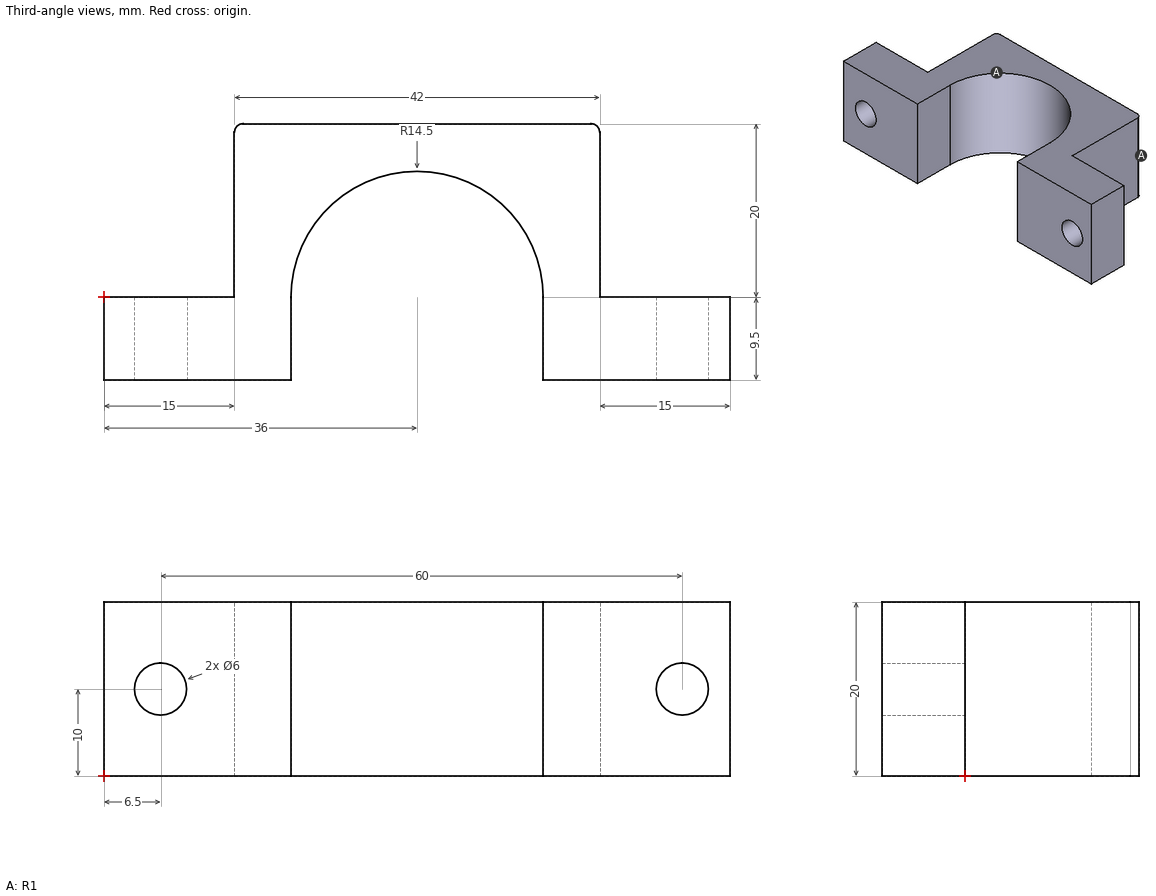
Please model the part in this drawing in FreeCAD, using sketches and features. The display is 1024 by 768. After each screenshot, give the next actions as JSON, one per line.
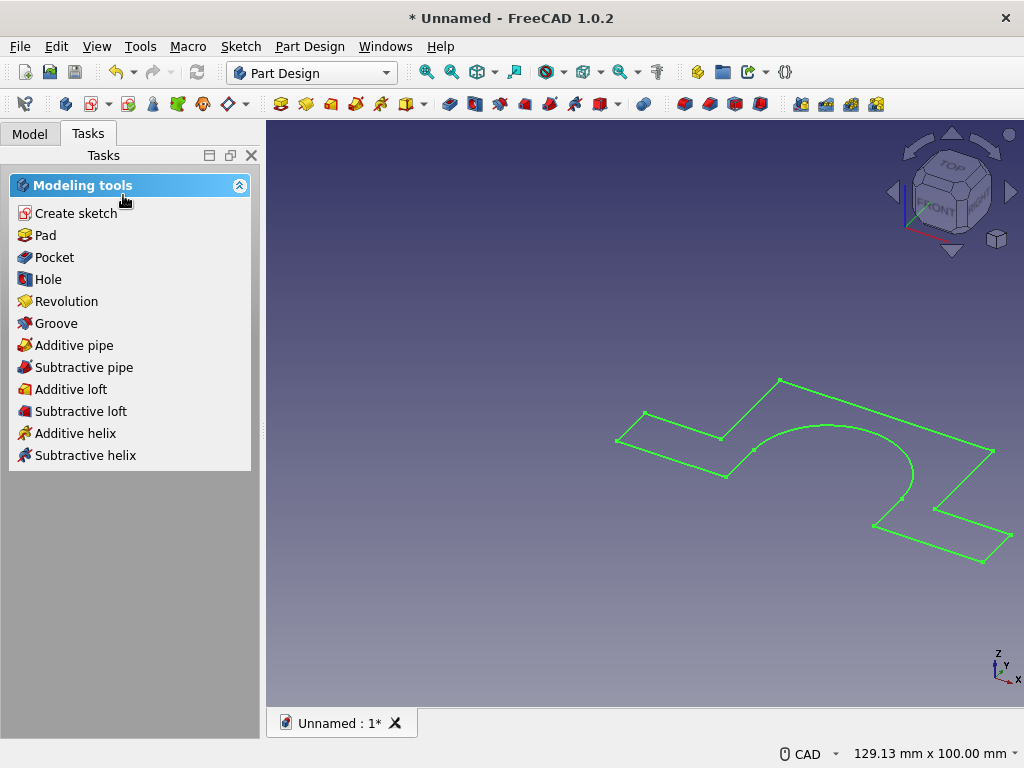
{"action": "left_click", "coordinate": [281, 104]}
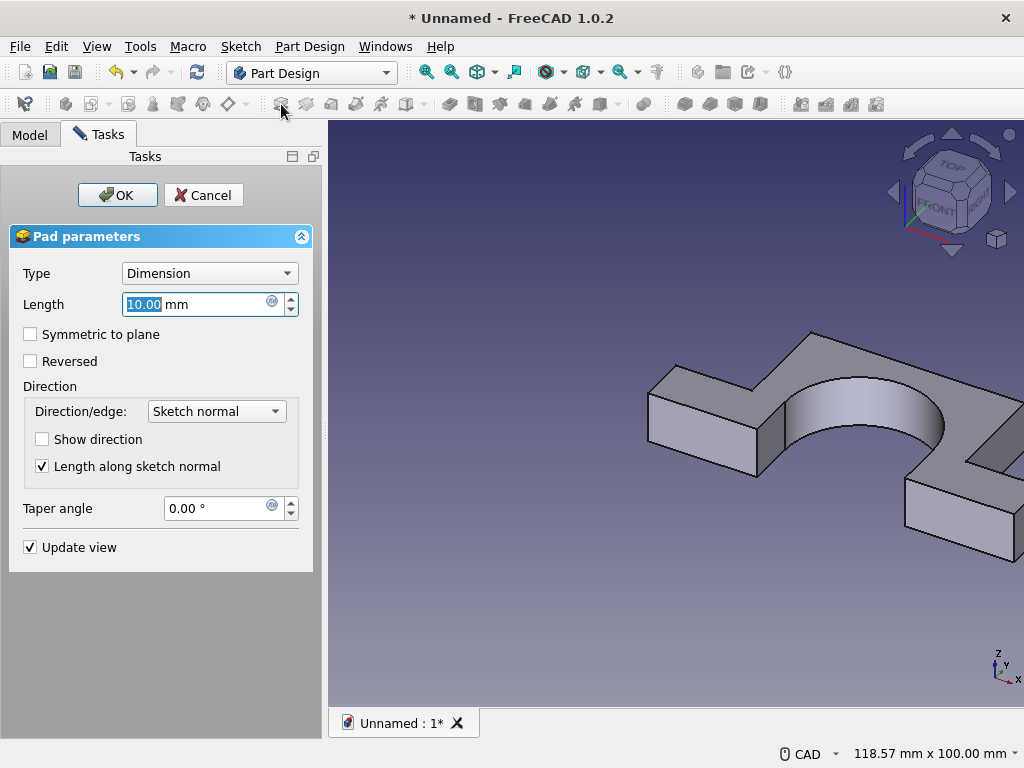
{"action": "type", "text": "20"}
{"action": "key", "text": "Tab"}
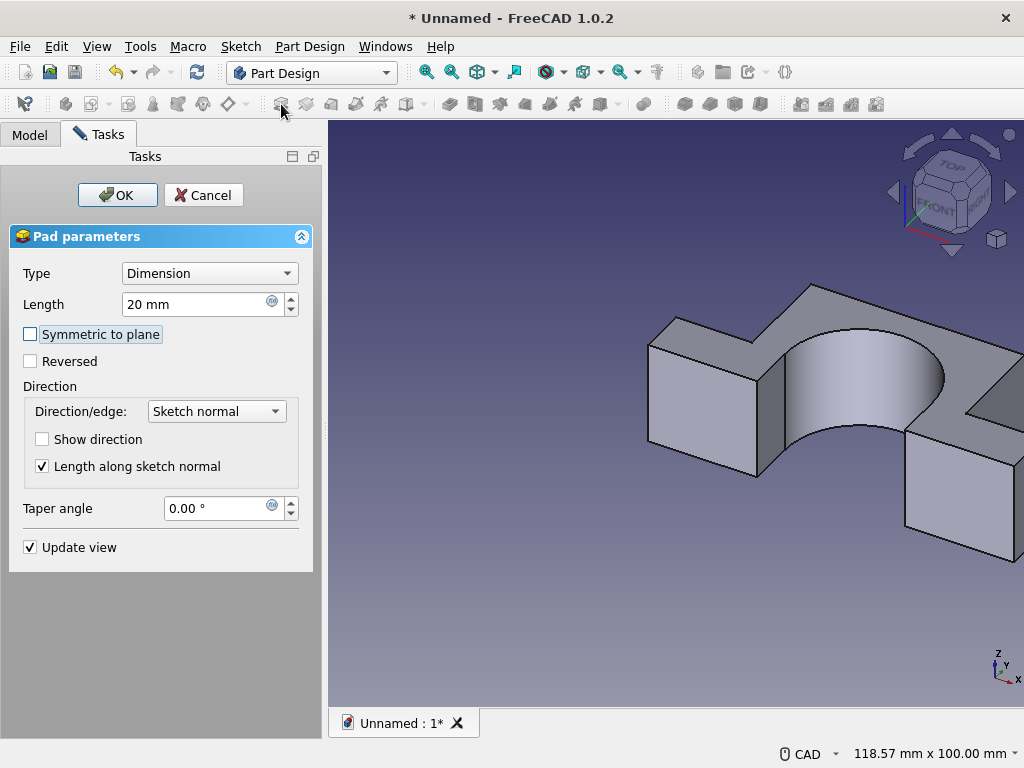
{"action": "left_click", "coordinate": [118, 195]}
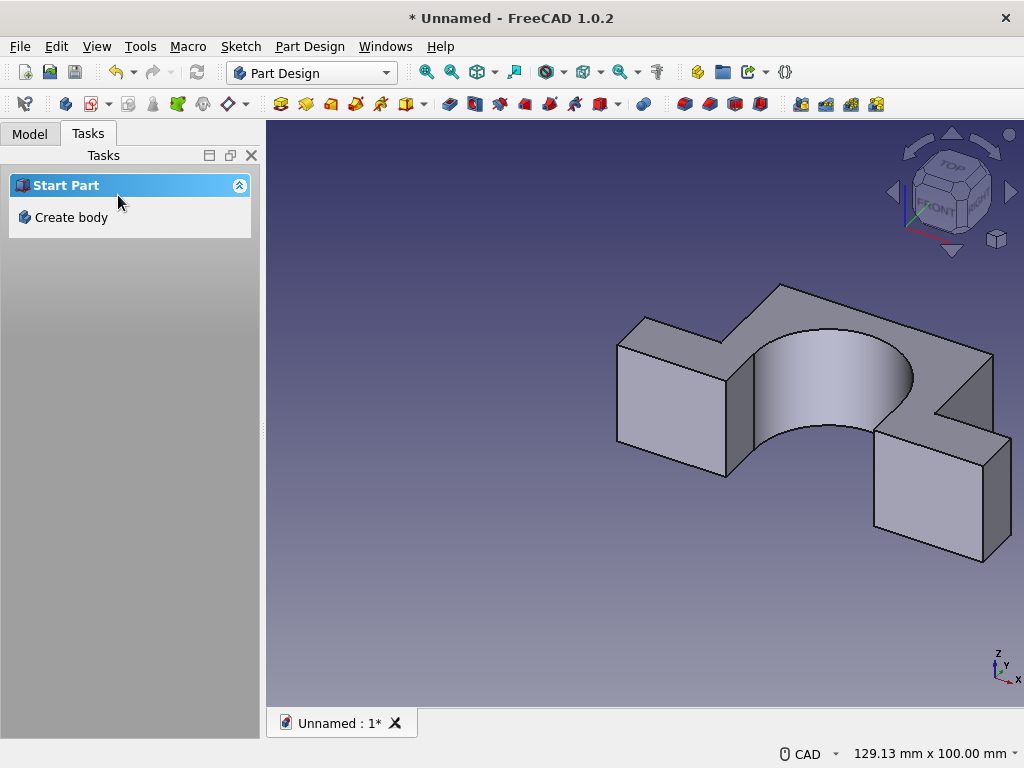
{"action": "left_click", "coordinate": [427, 72]}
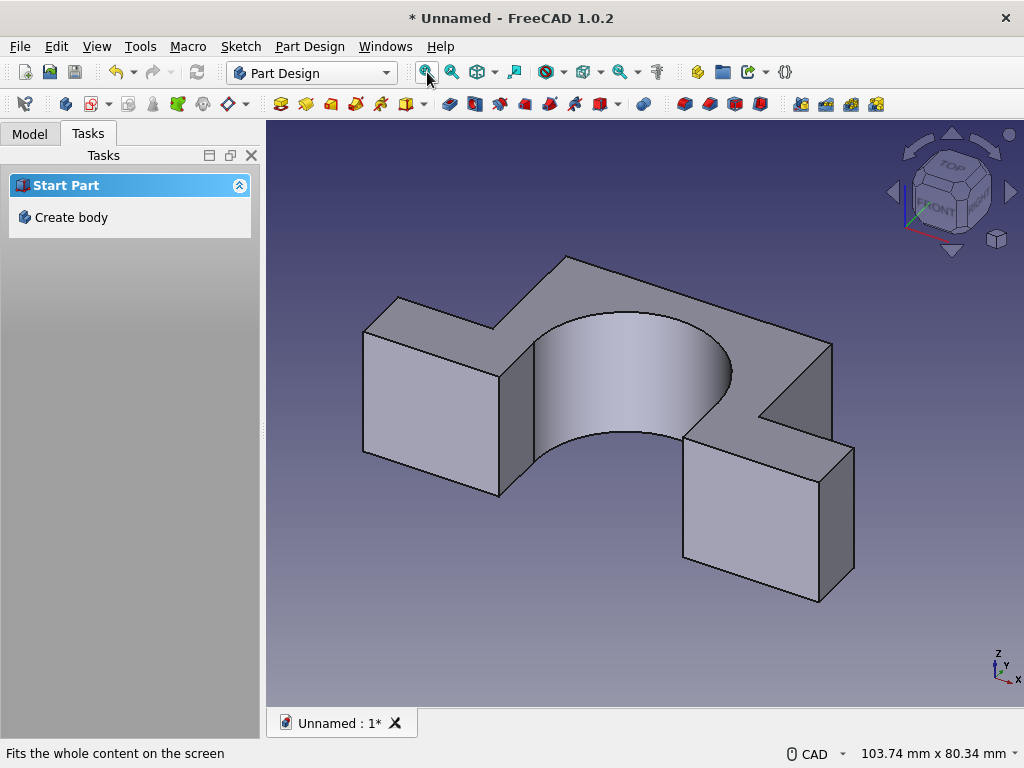
{"action": "key", "text": "0"}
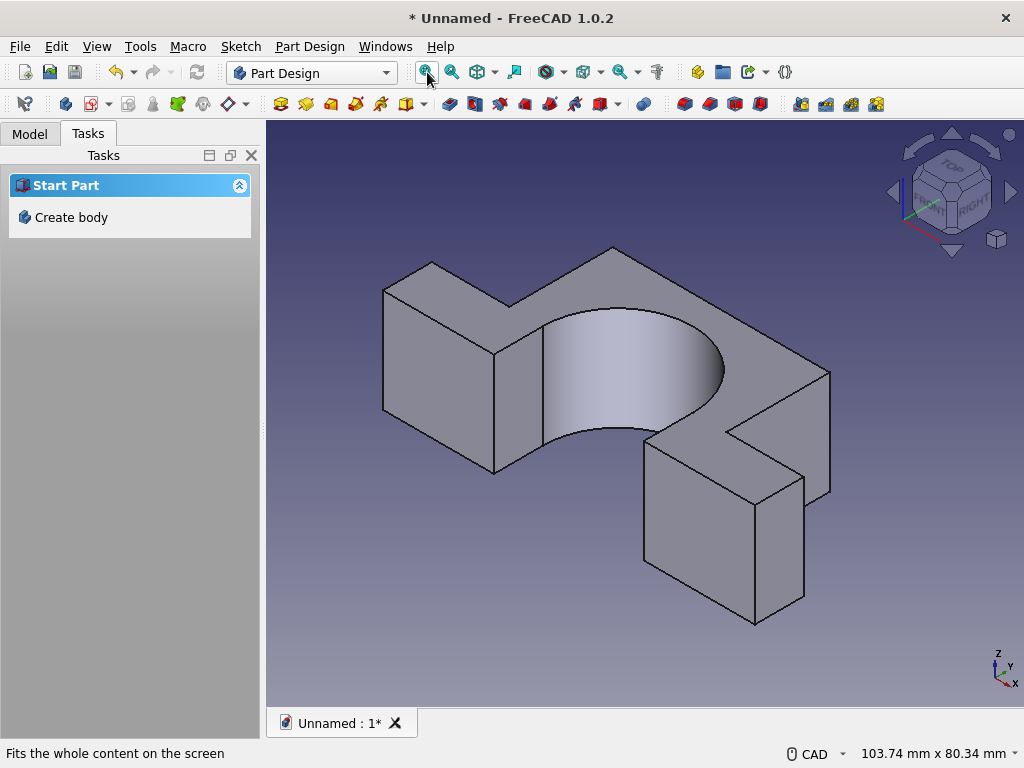
{"action": "key", "text": "2"}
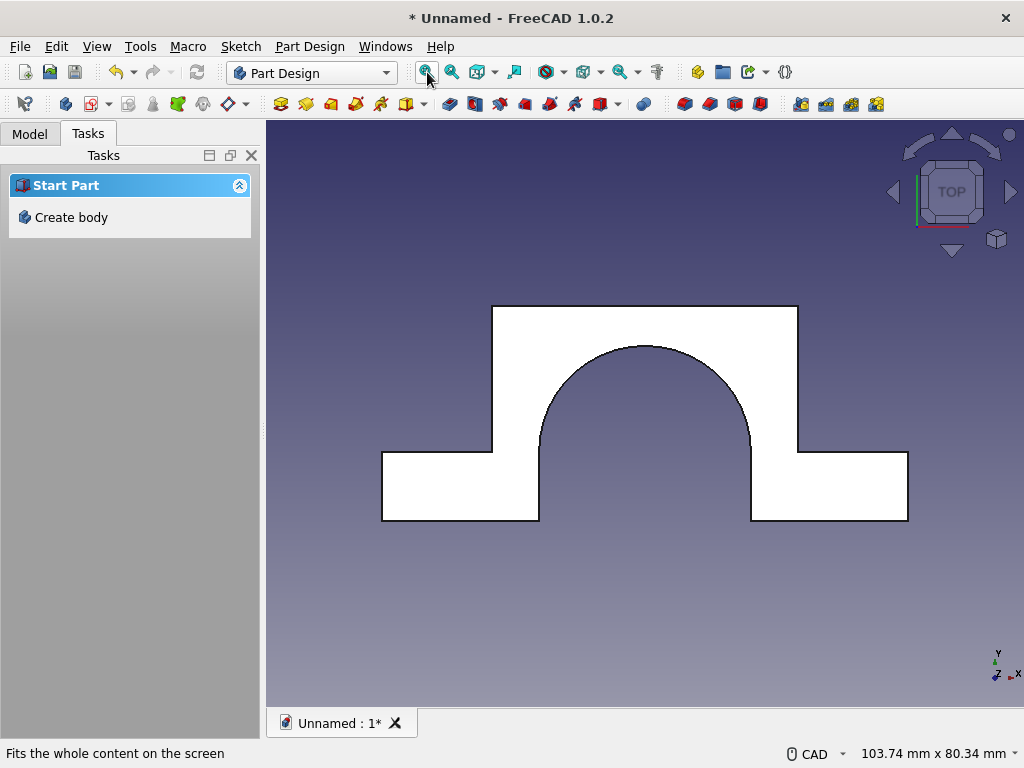
{"action": "key", "text": "1"}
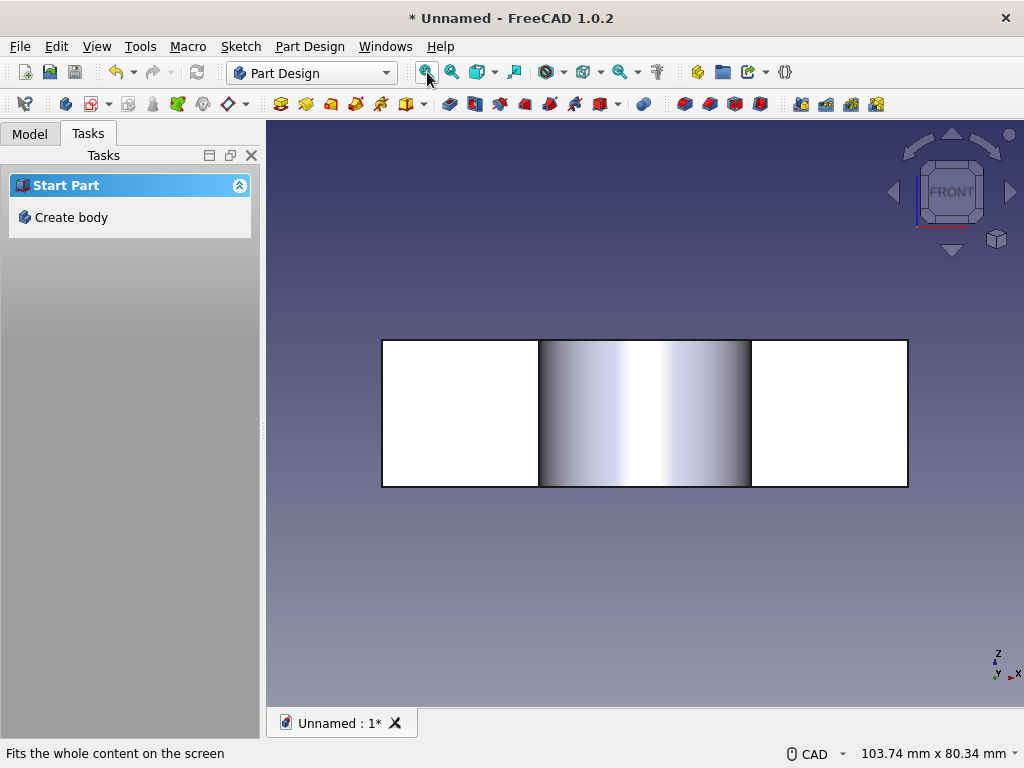
{"action": "key", "text": "3"}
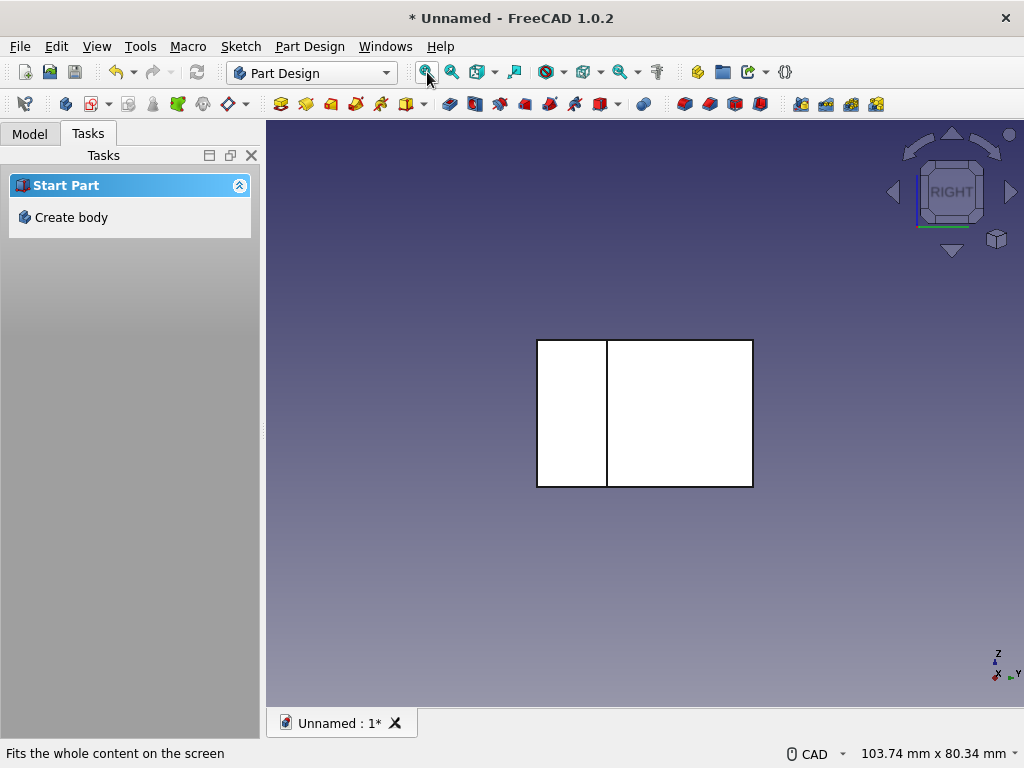
{"action": "left_click", "coordinate": [427, 72]}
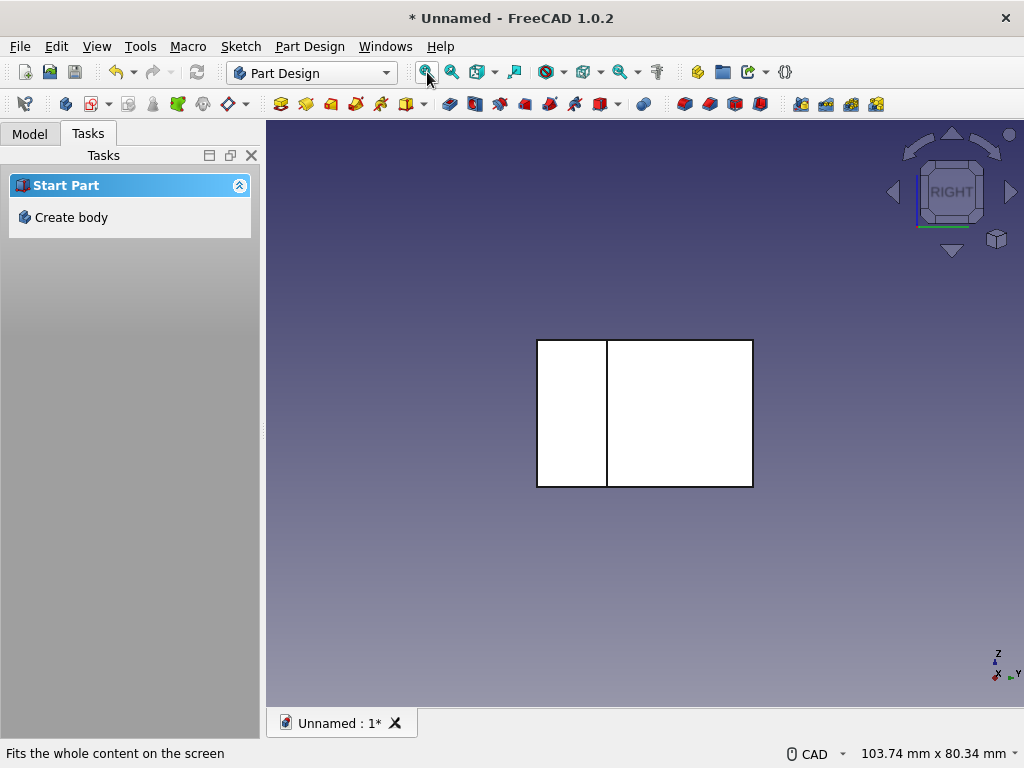
{"action": "left_click", "coordinate": [753, 412]}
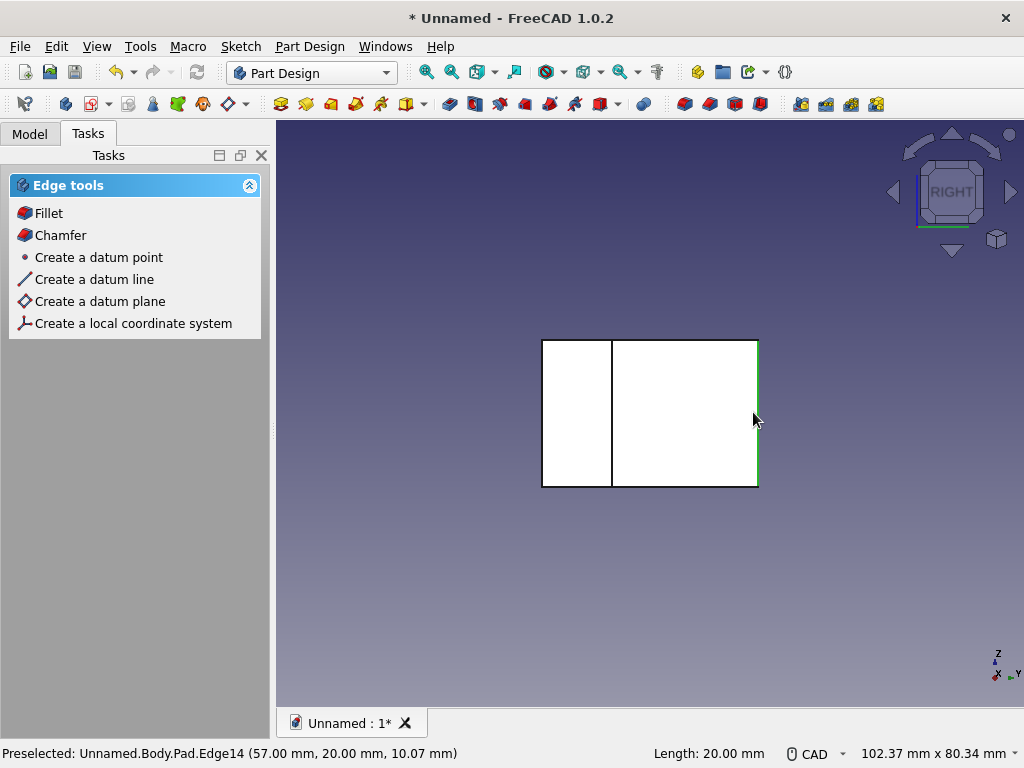
{"action": "key", "text": "5"}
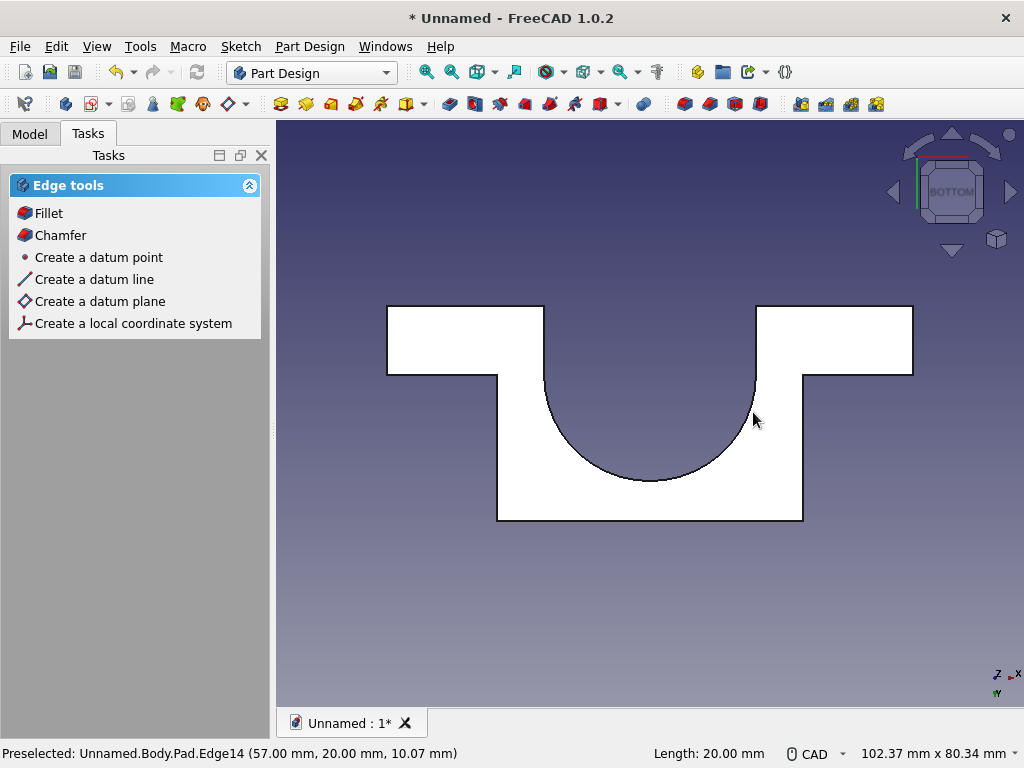
{"action": "key", "text": "4"}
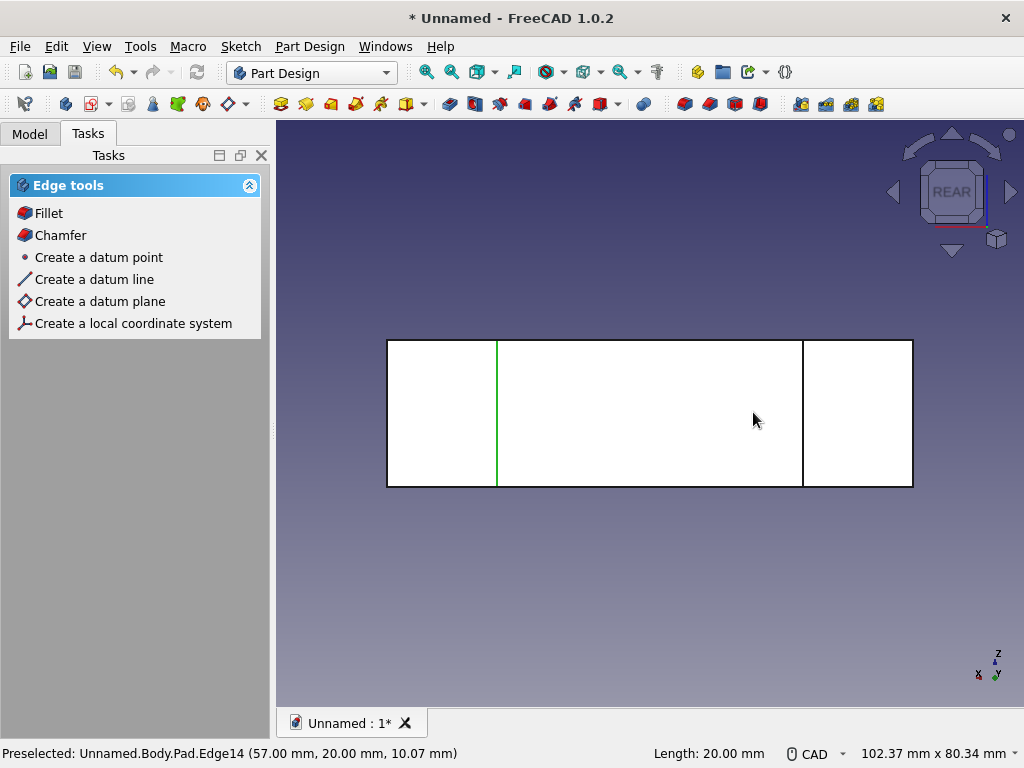
{"action": "left_click", "coordinate": [803, 413], "text": "ctrl"}